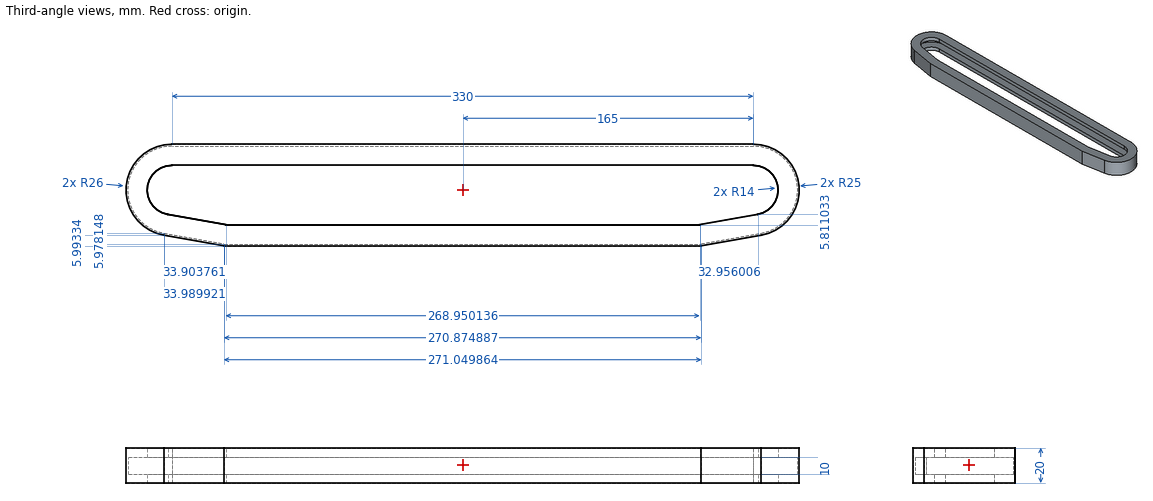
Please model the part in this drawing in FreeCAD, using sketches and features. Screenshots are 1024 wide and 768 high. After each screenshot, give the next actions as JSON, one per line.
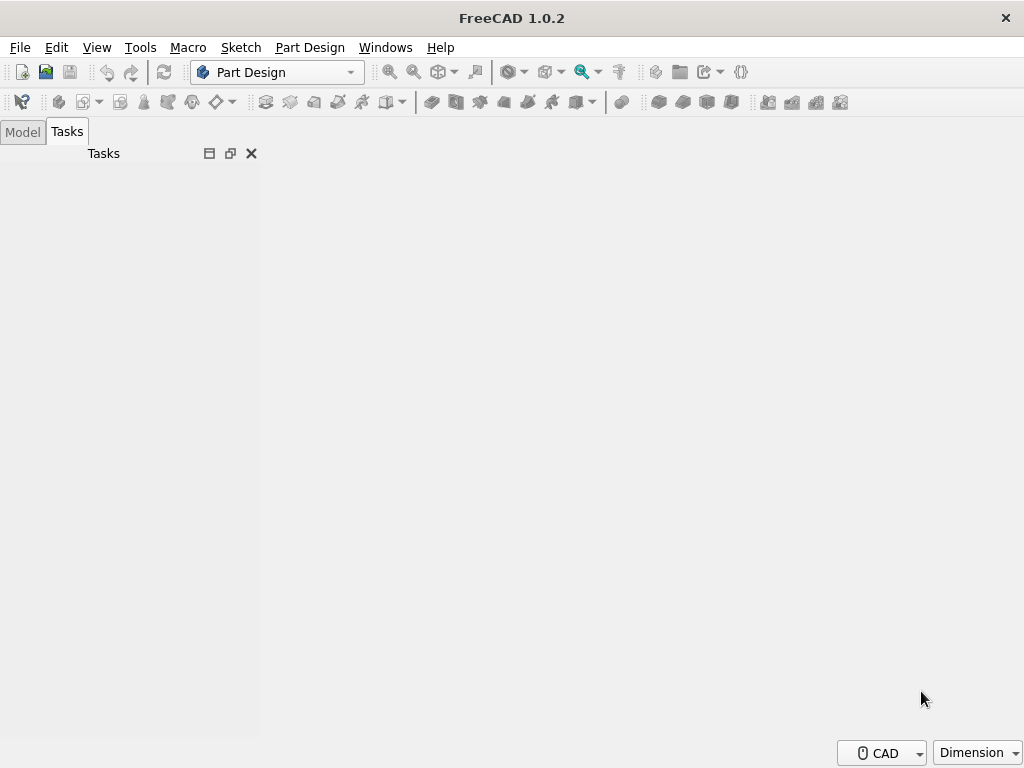
{"action": "left_click", "coordinate": [22, 72]}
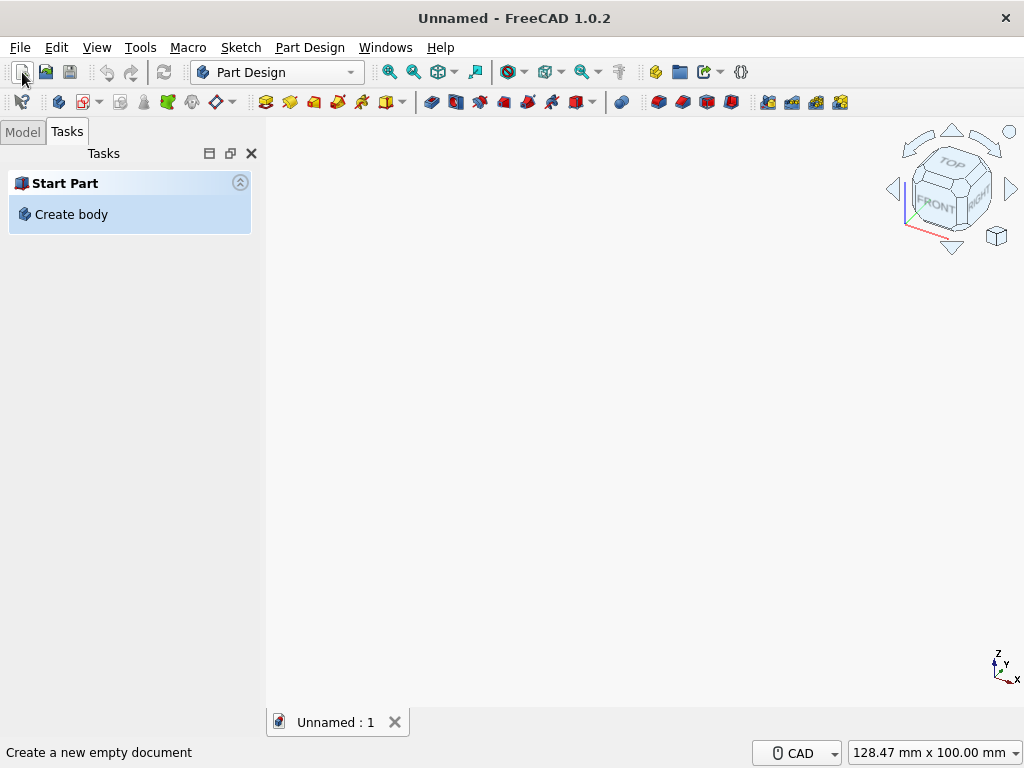
{"action": "left_click", "coordinate": [84, 102]}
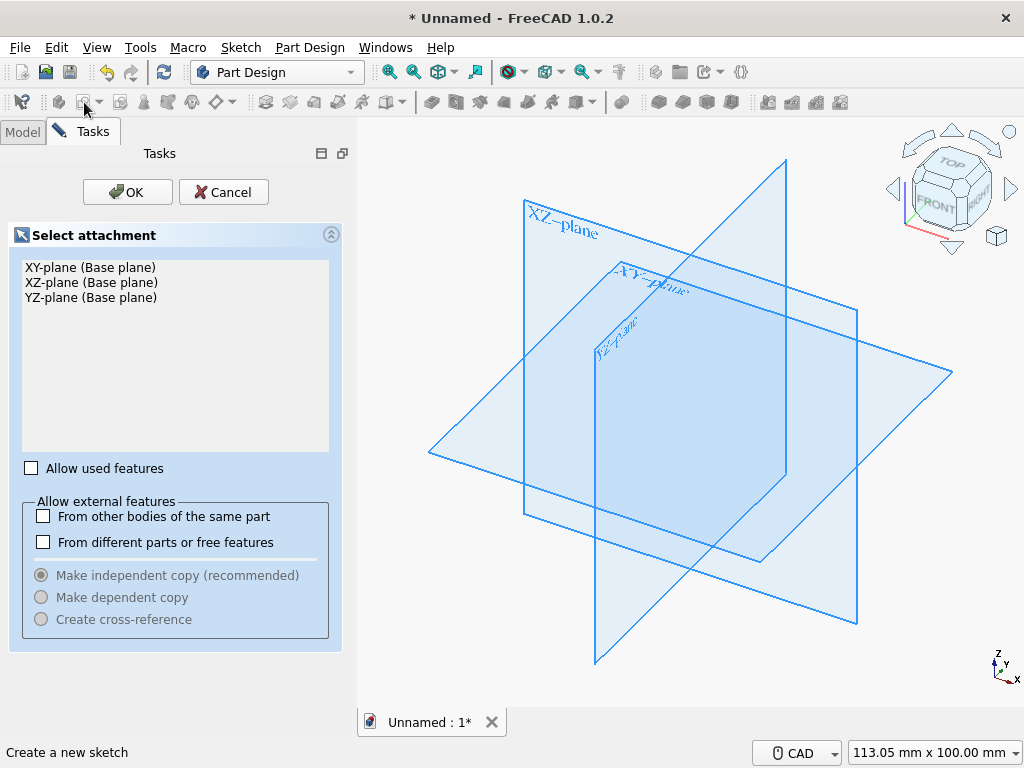
{"action": "left_click", "coordinate": [82, 268]}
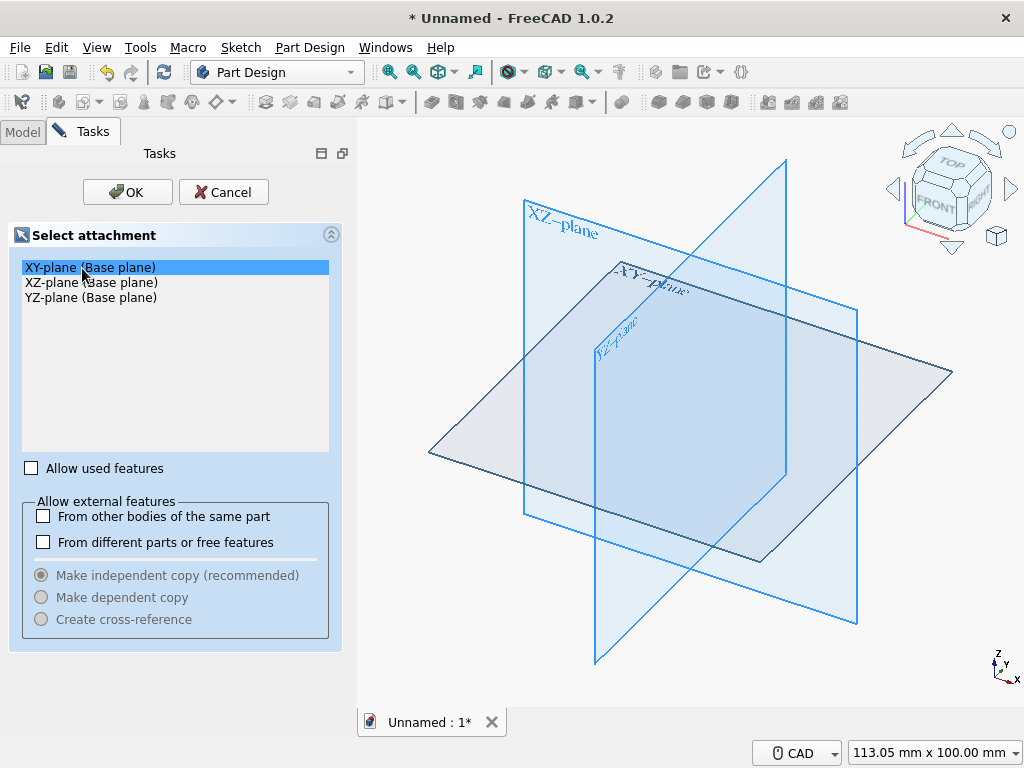
{"action": "left_click", "coordinate": [128, 192]}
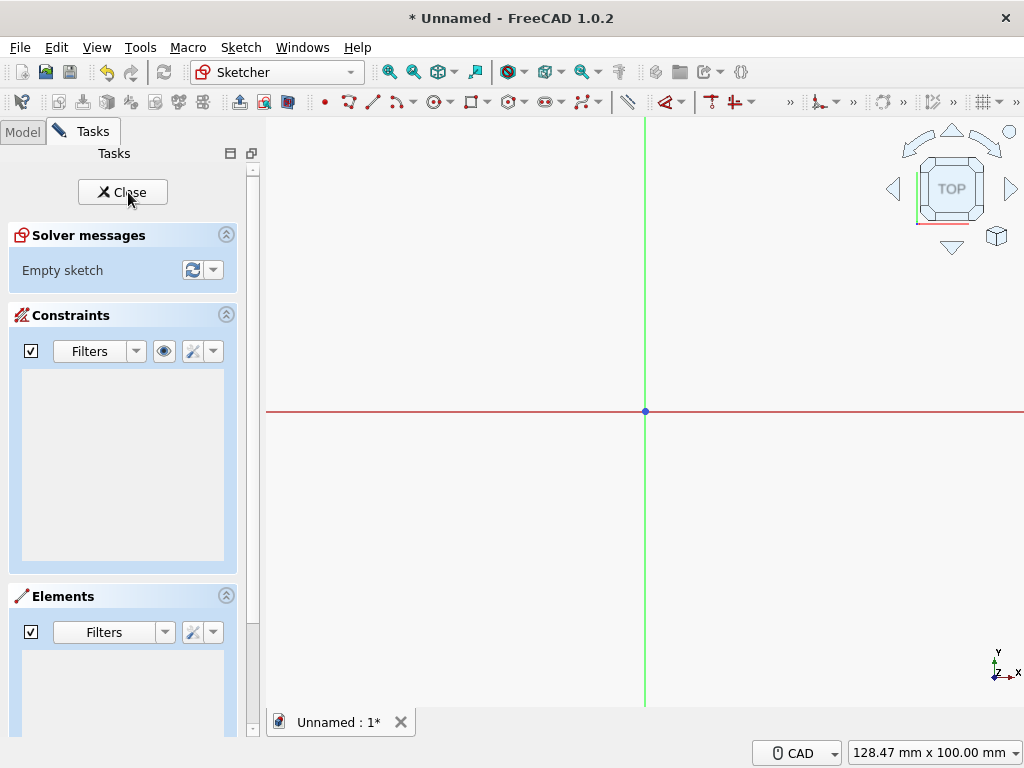
{"action": "scroll", "coordinate": [563, 409], "scroll_direction": "down", "scroll_amount": 9}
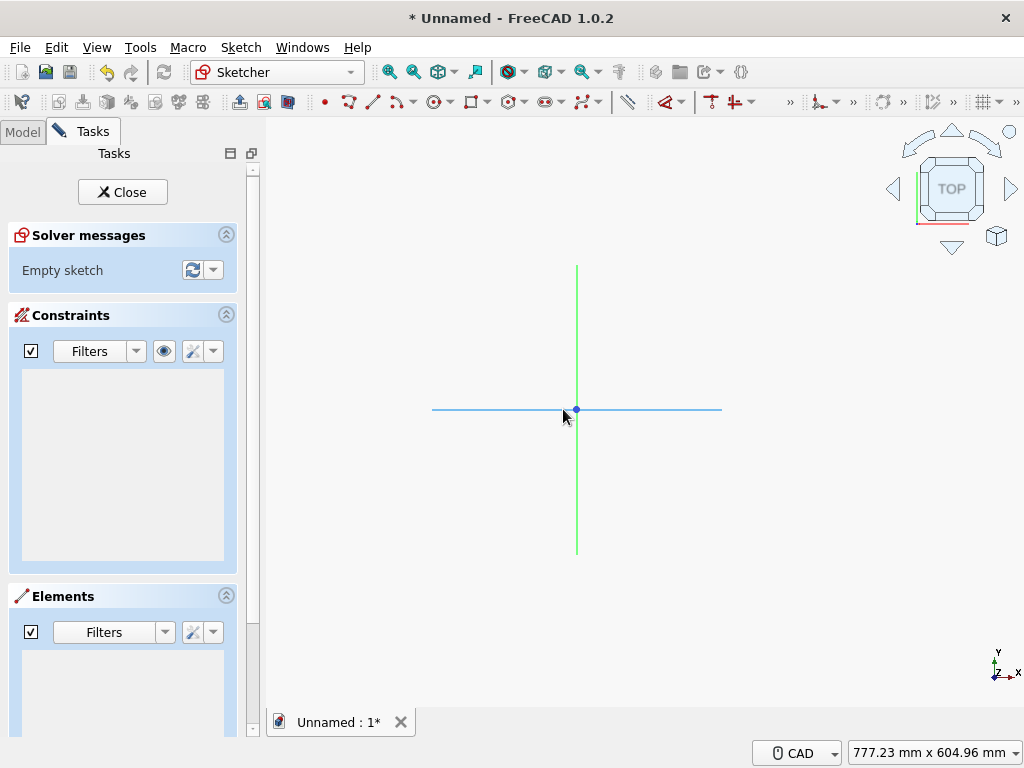
{"action": "left_click", "coordinate": [374, 102]}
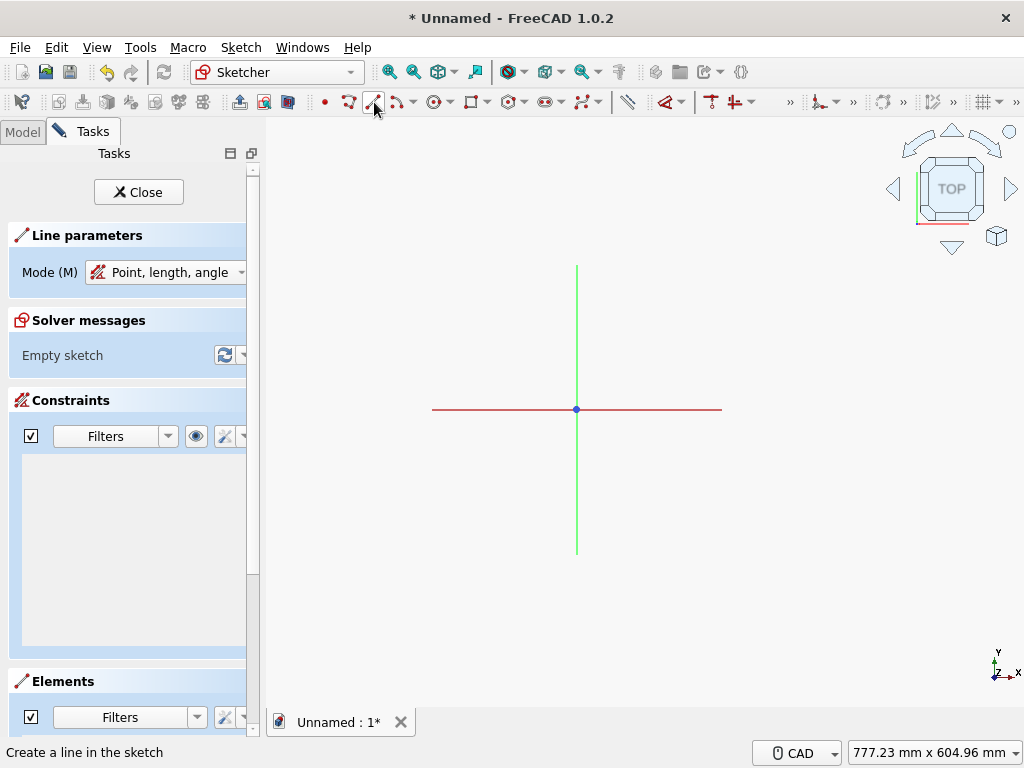
{"action": "left_click", "coordinate": [738, 385]}
{"action": "left_click", "coordinate": [416, 385]}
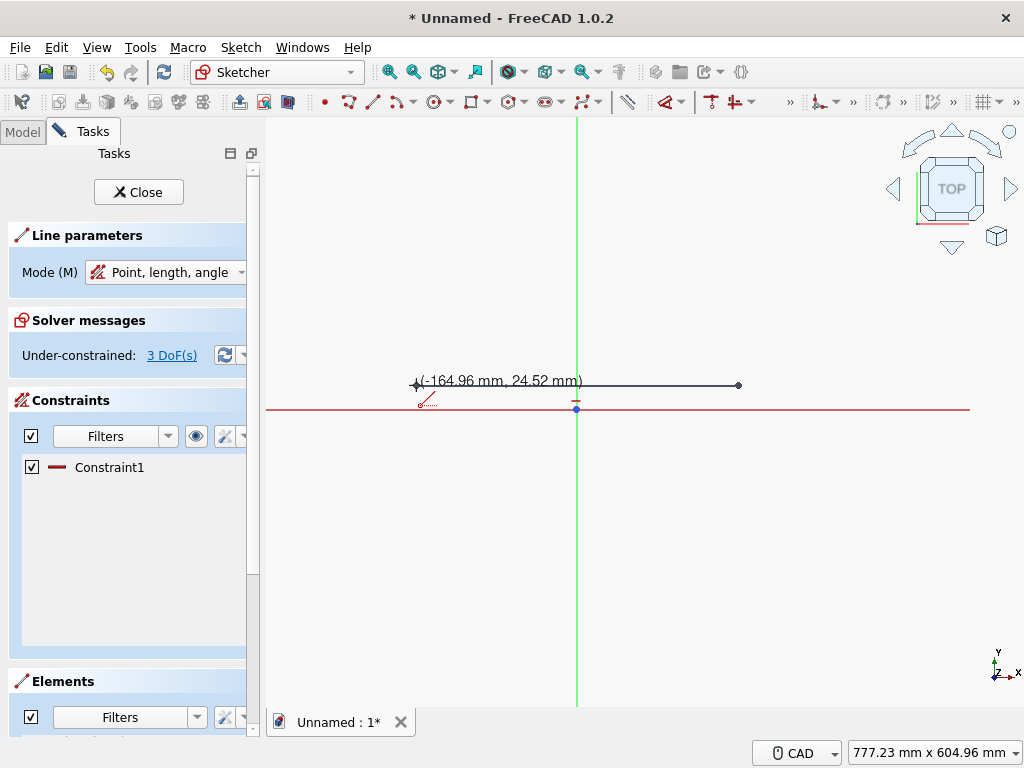
{"action": "left_click", "coordinate": [350, 102]}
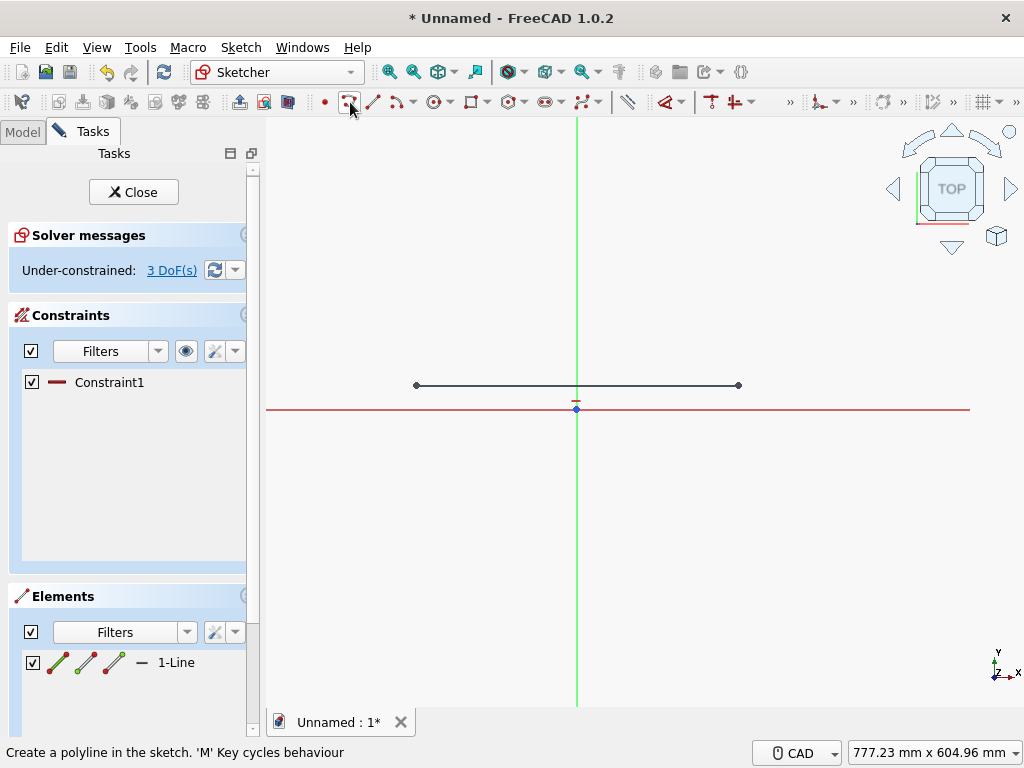
{"action": "left_click", "coordinate": [412, 435]}
{"action": "left_click", "coordinate": [445, 441]}
{"action": "left_click", "coordinate": [709, 441]}
{"action": "left_click", "coordinate": [742, 435]}
{"action": "right_click", "coordinate": [742, 435]}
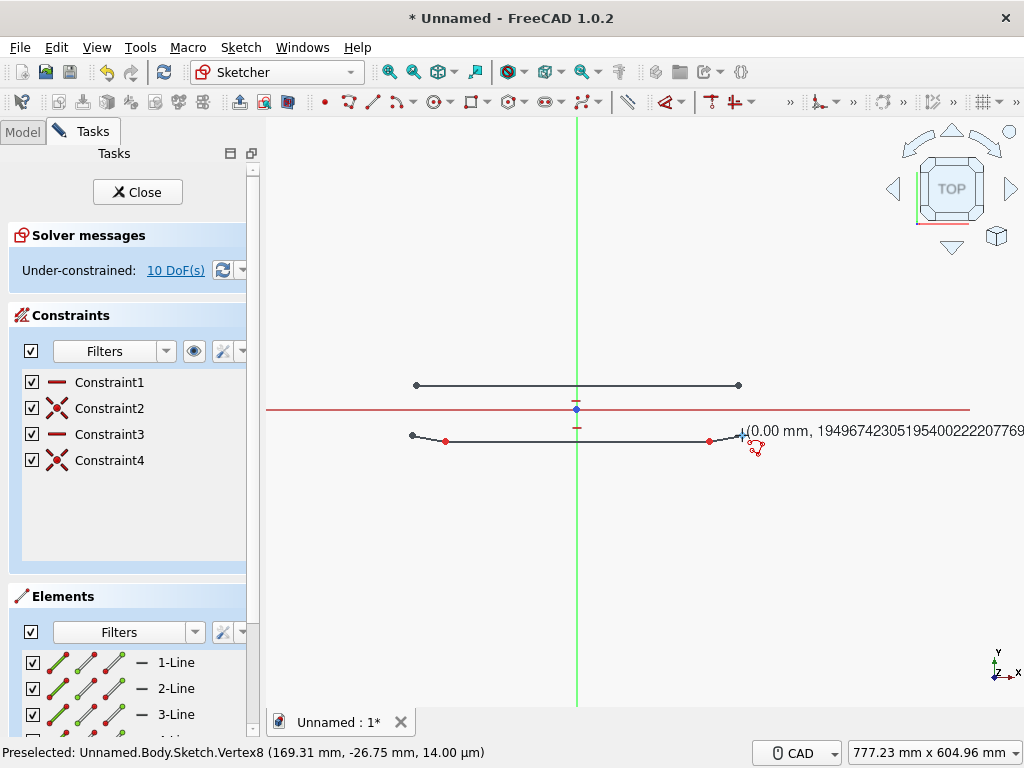
{"action": "left_click", "coordinate": [416, 102]}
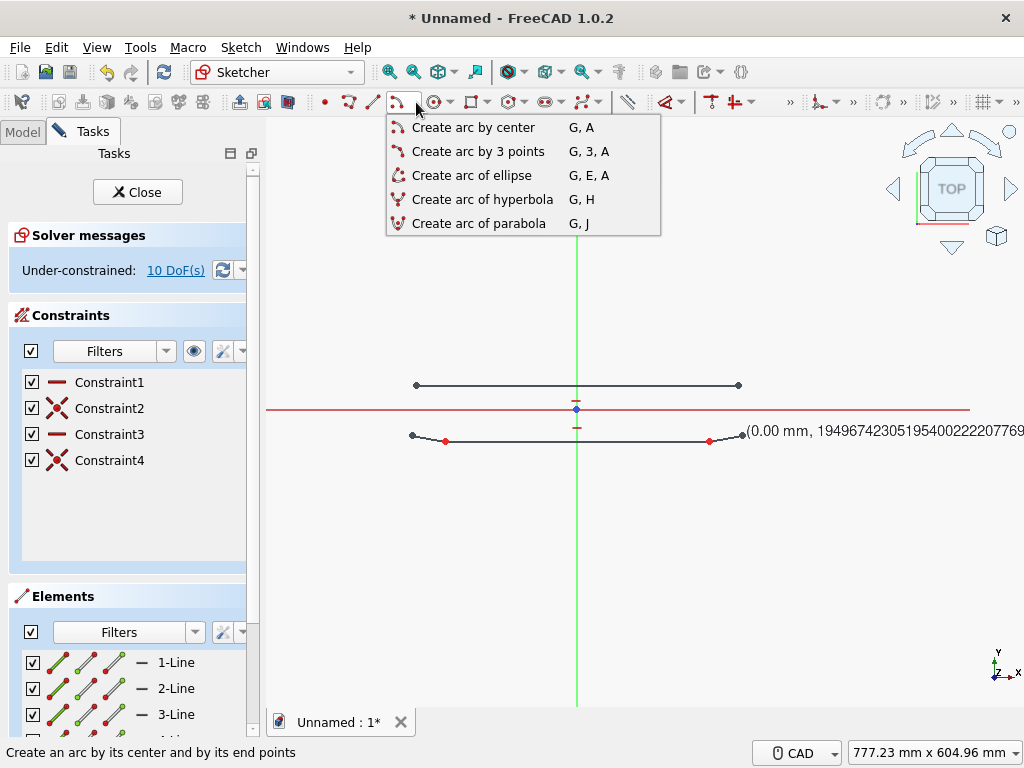
{"action": "left_click", "coordinate": [524, 151]}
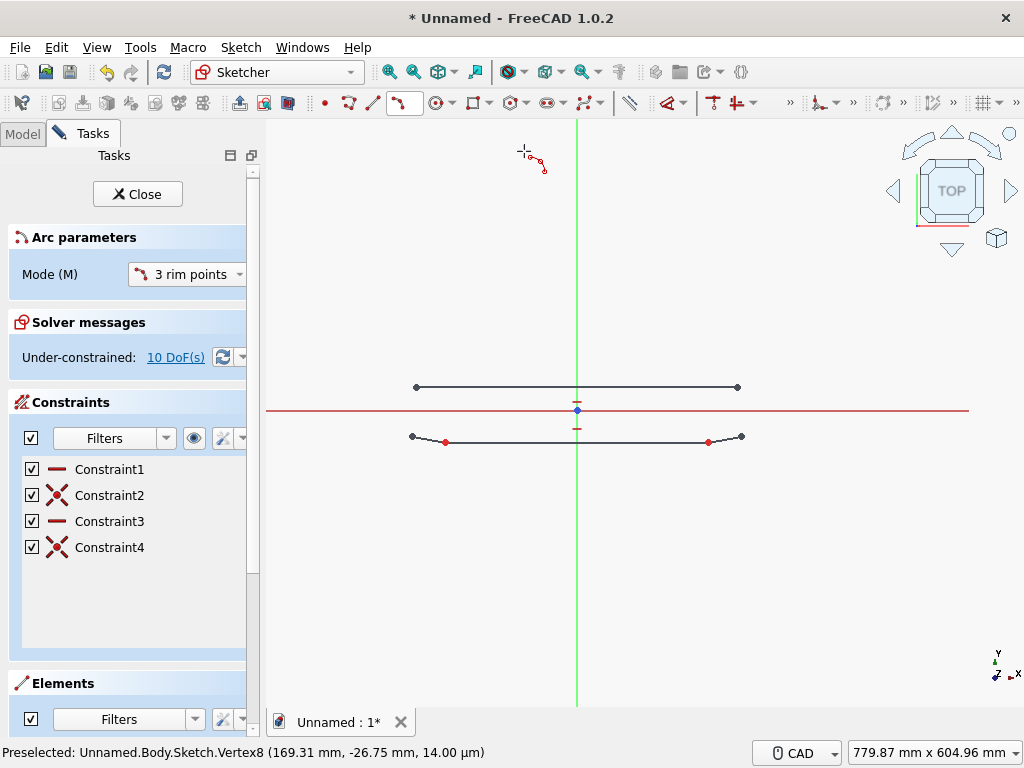
{"action": "left_click", "coordinate": [417, 387]}
{"action": "left_click", "coordinate": [413, 437]}
{"action": "left_click", "coordinate": [397, 395]}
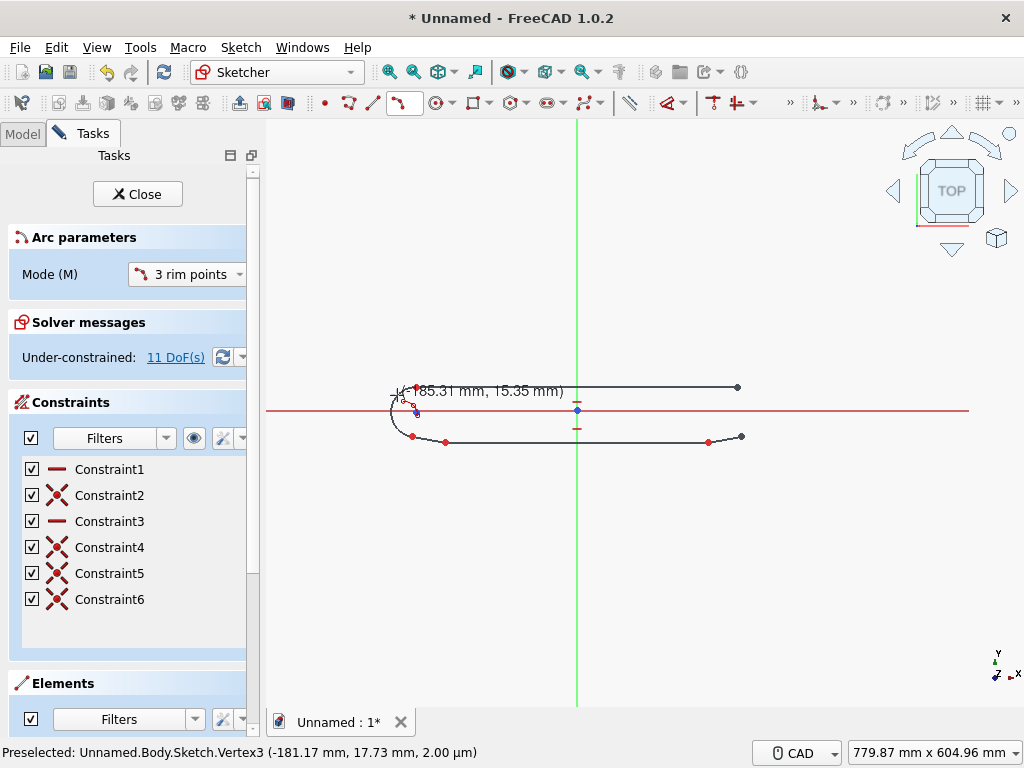
{"action": "left_click", "coordinate": [742, 437]}
{"action": "left_click", "coordinate": [738, 387]}
{"action": "left_click", "coordinate": [757, 395]}